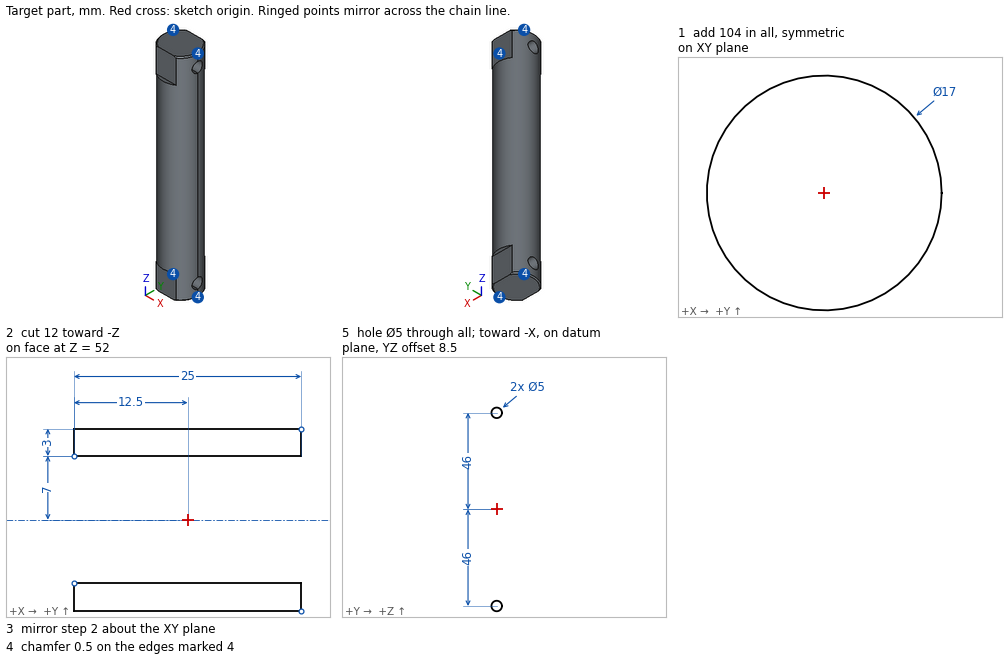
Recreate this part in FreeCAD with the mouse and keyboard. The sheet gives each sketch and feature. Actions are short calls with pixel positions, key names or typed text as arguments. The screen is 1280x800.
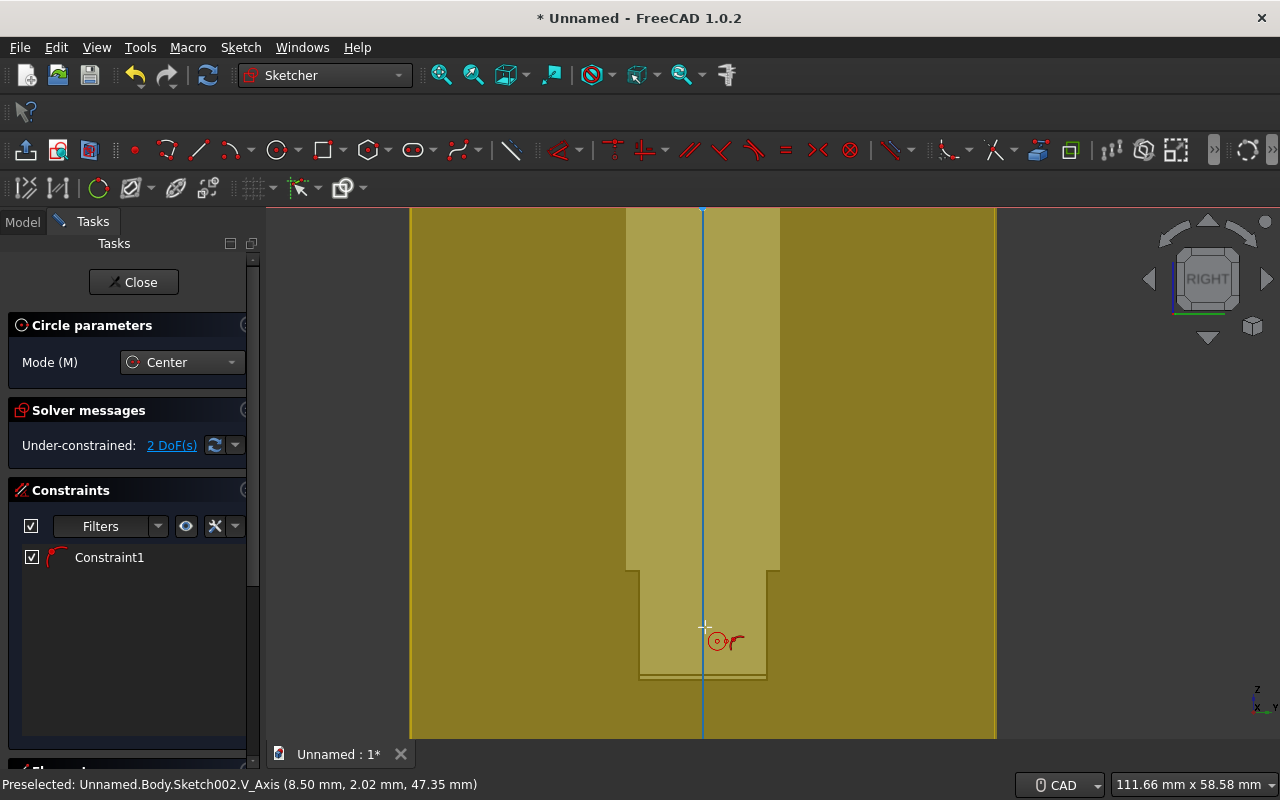
click(703, 625)
click(719, 609)
key(Escape)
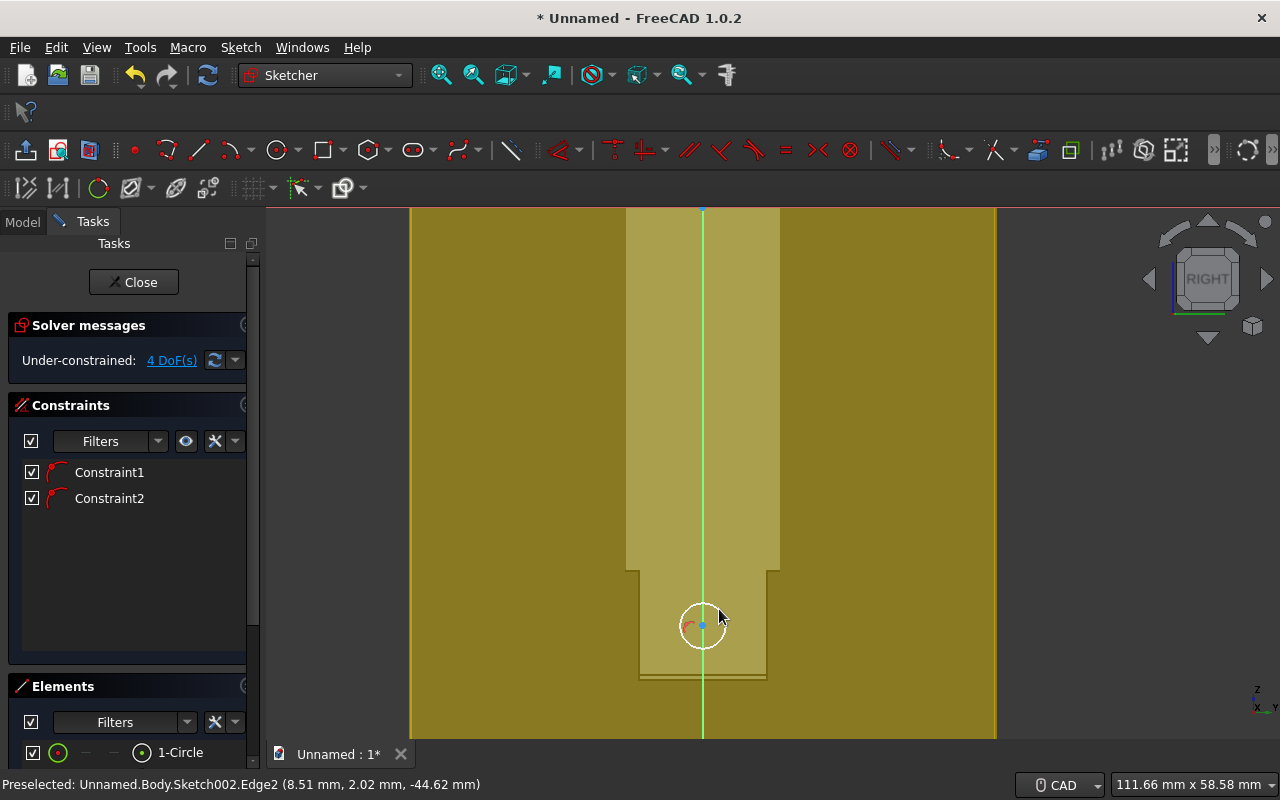
scroll(705, 628, down, 5)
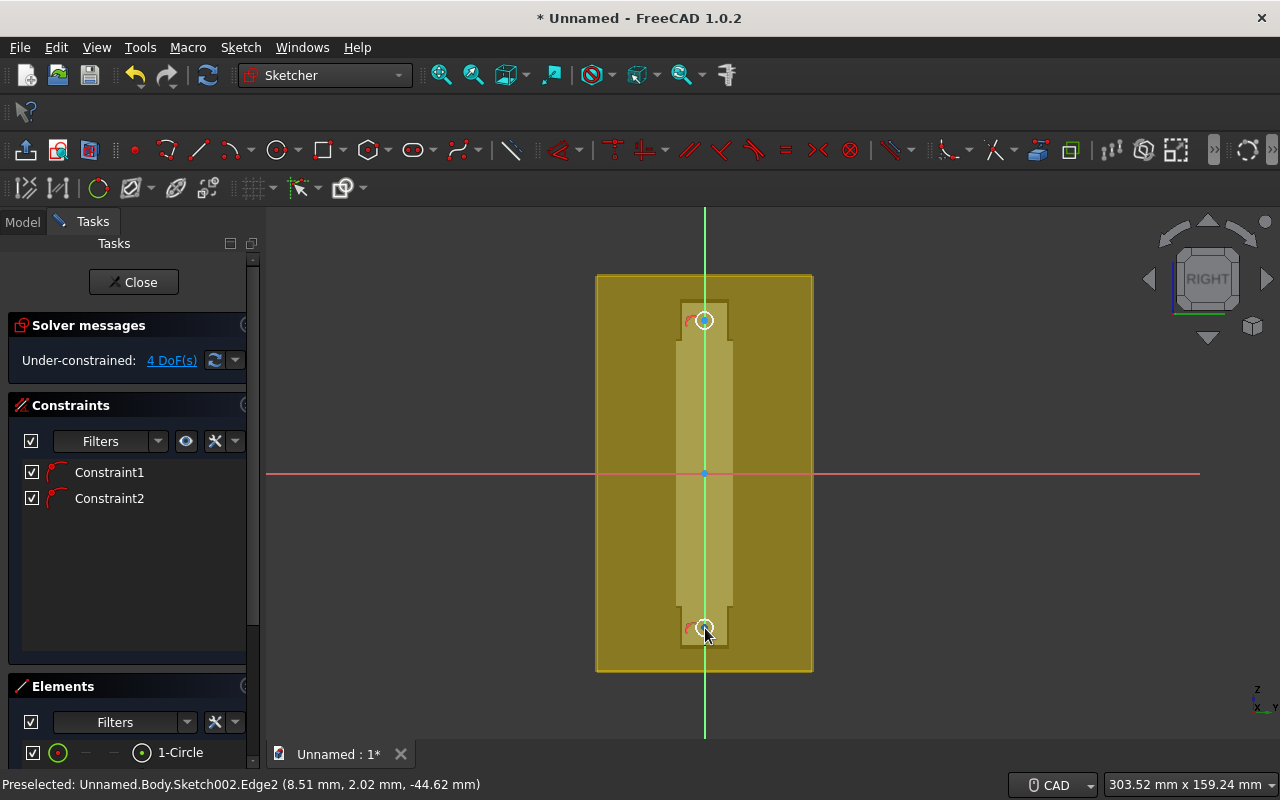
scroll(710, 315, up, 5)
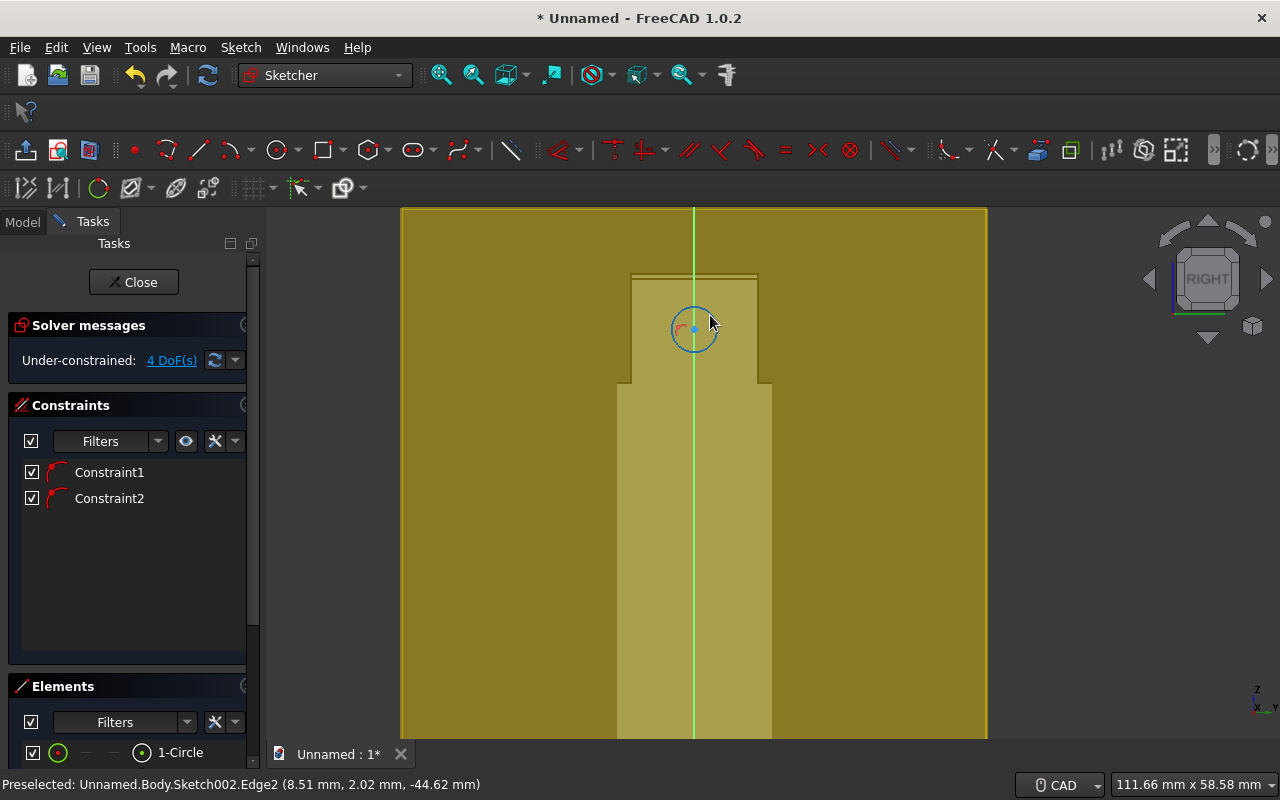
click(710, 314)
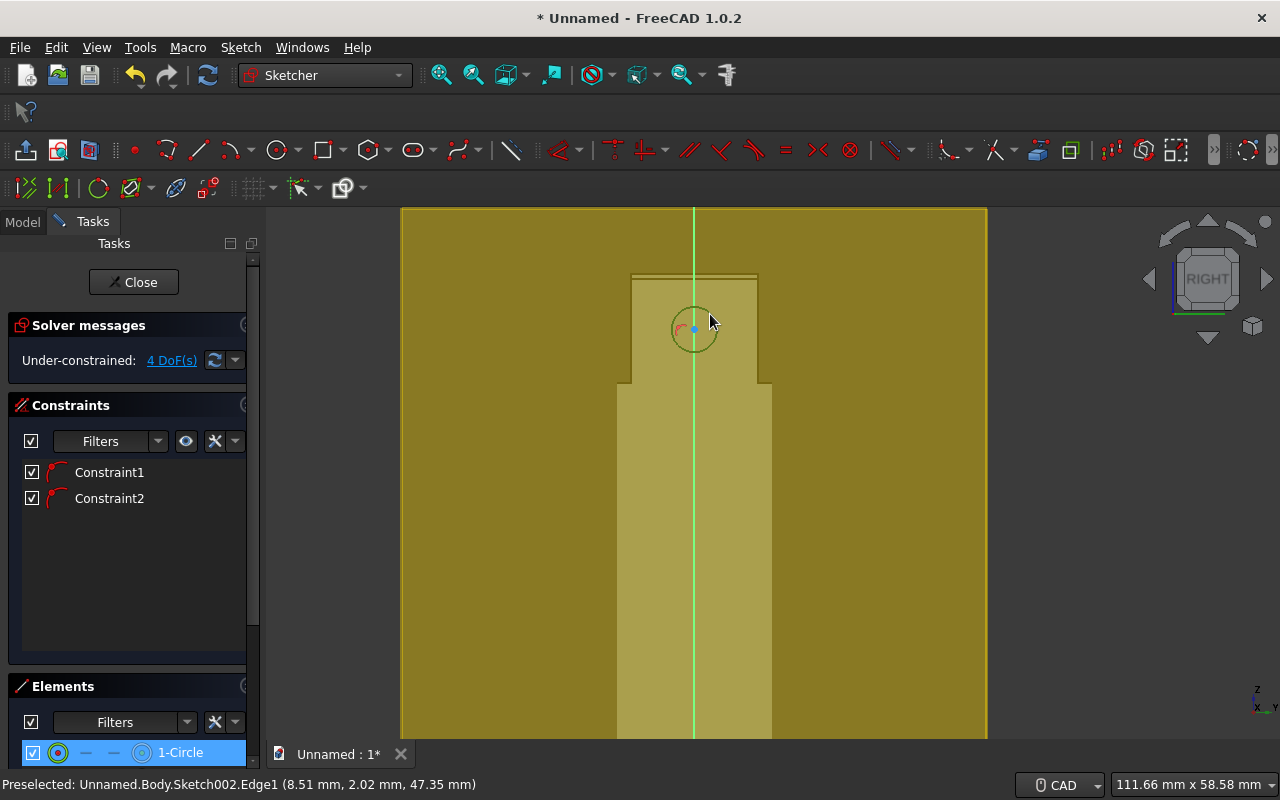
scroll(710, 314, down, 5)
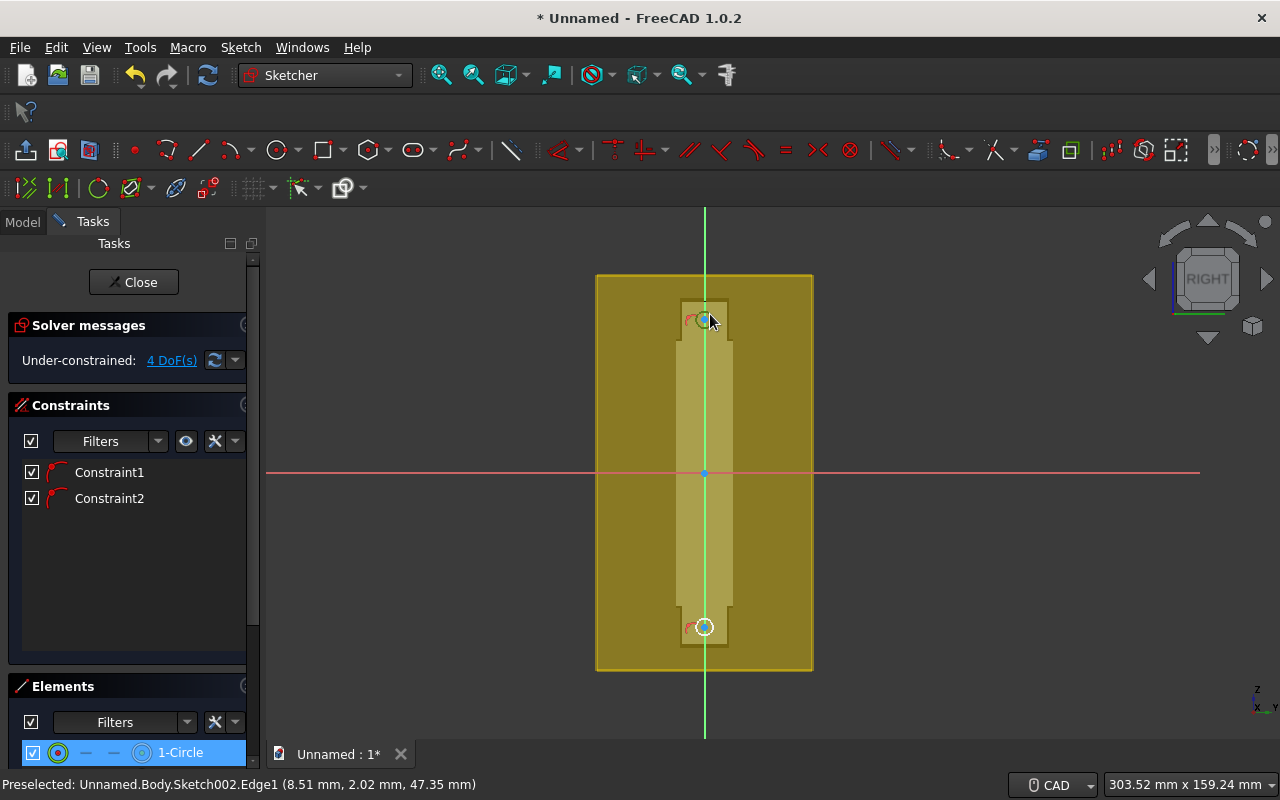
scroll(710, 621, up, 5)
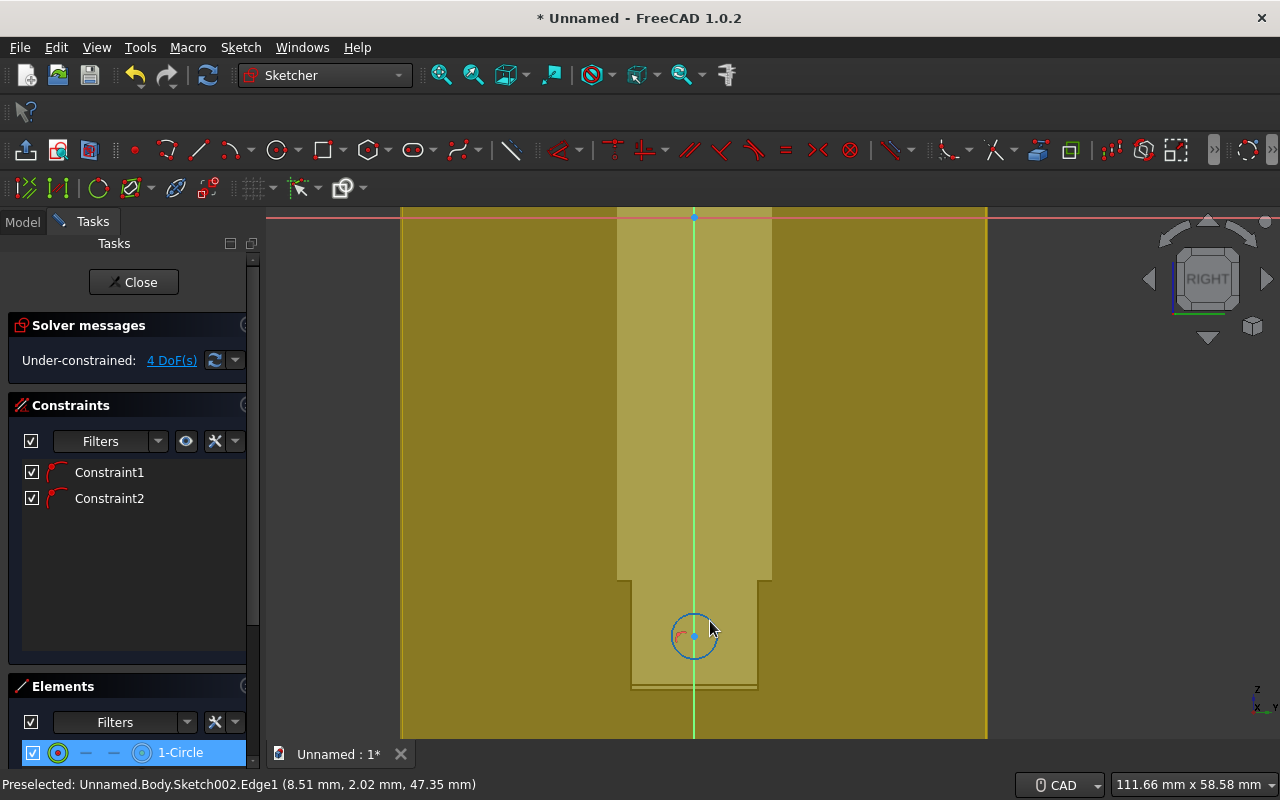
click(710, 620)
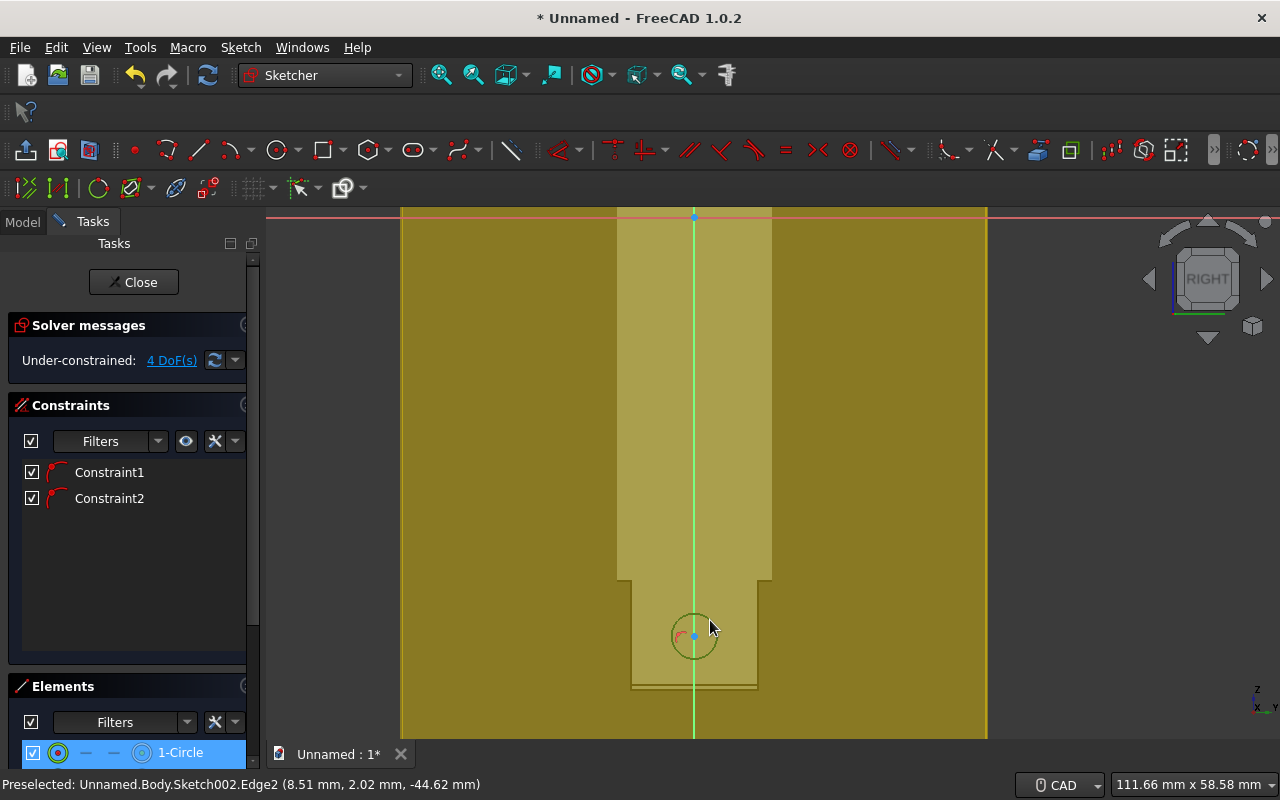
click(786, 150)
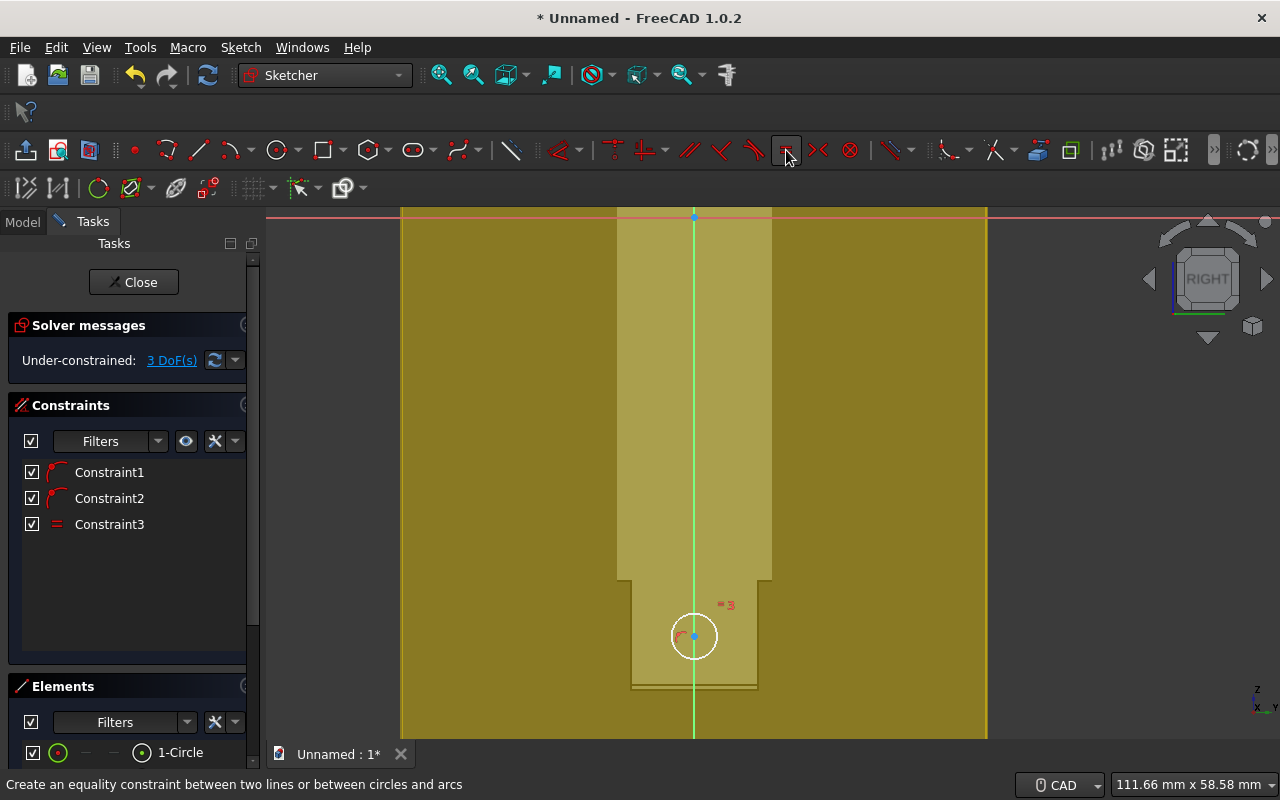
click(558, 150)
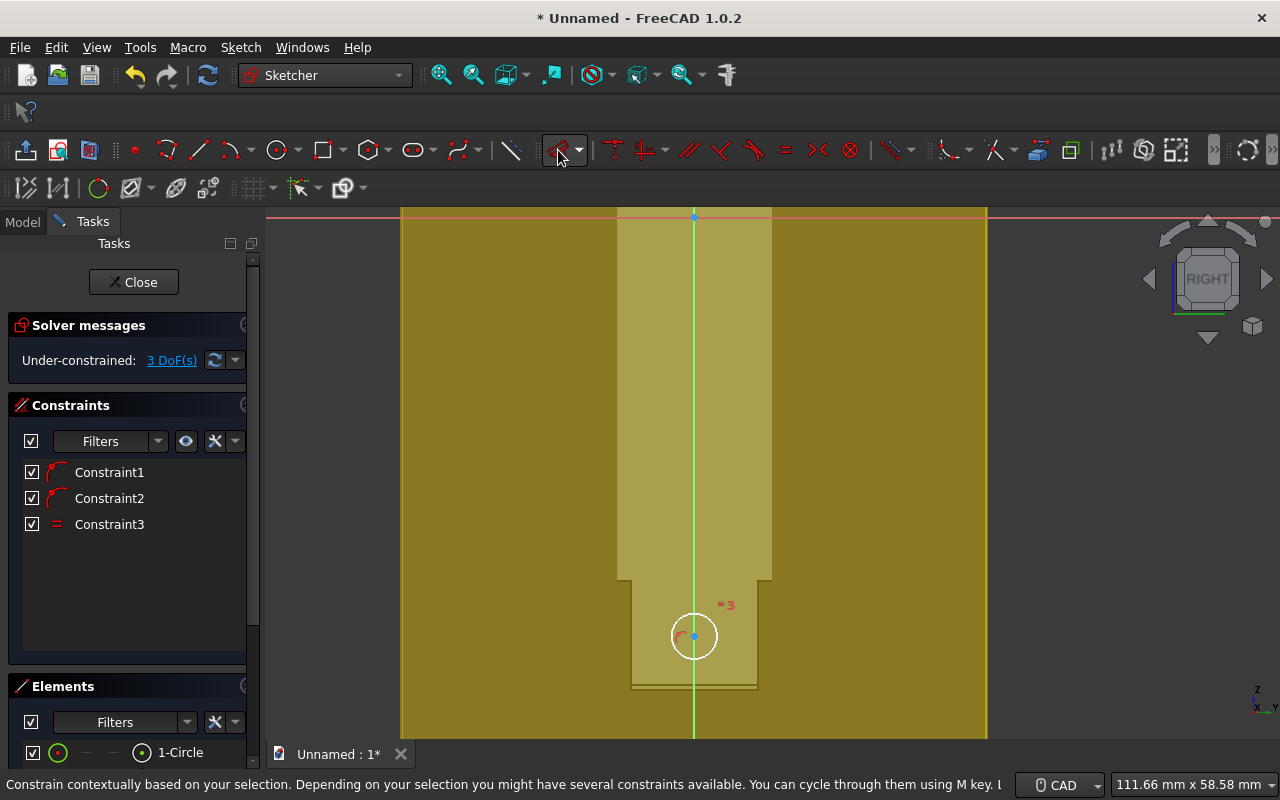
scroll(710, 622, down, 5)